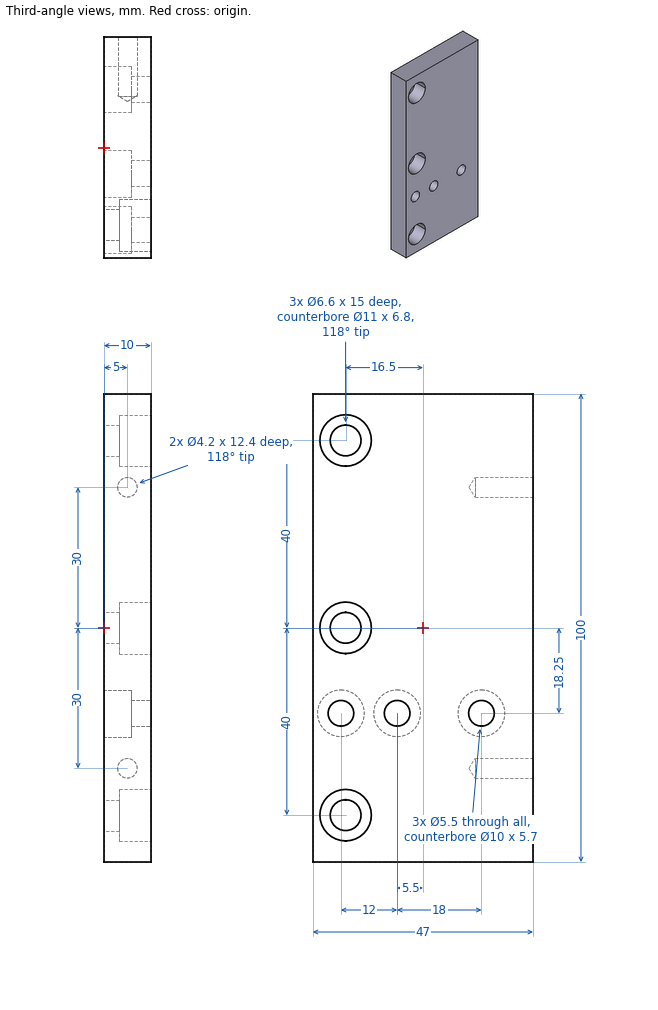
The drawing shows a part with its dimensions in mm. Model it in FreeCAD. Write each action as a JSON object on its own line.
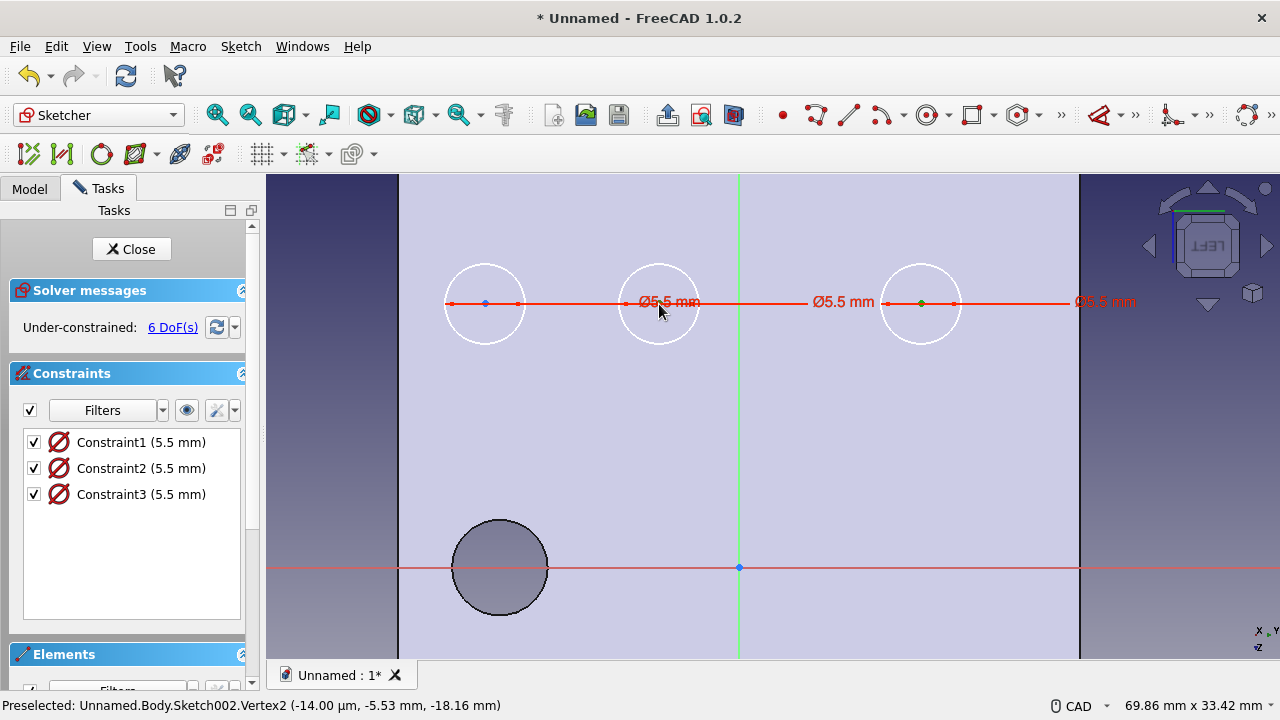
{"action": "key", "text": "h"}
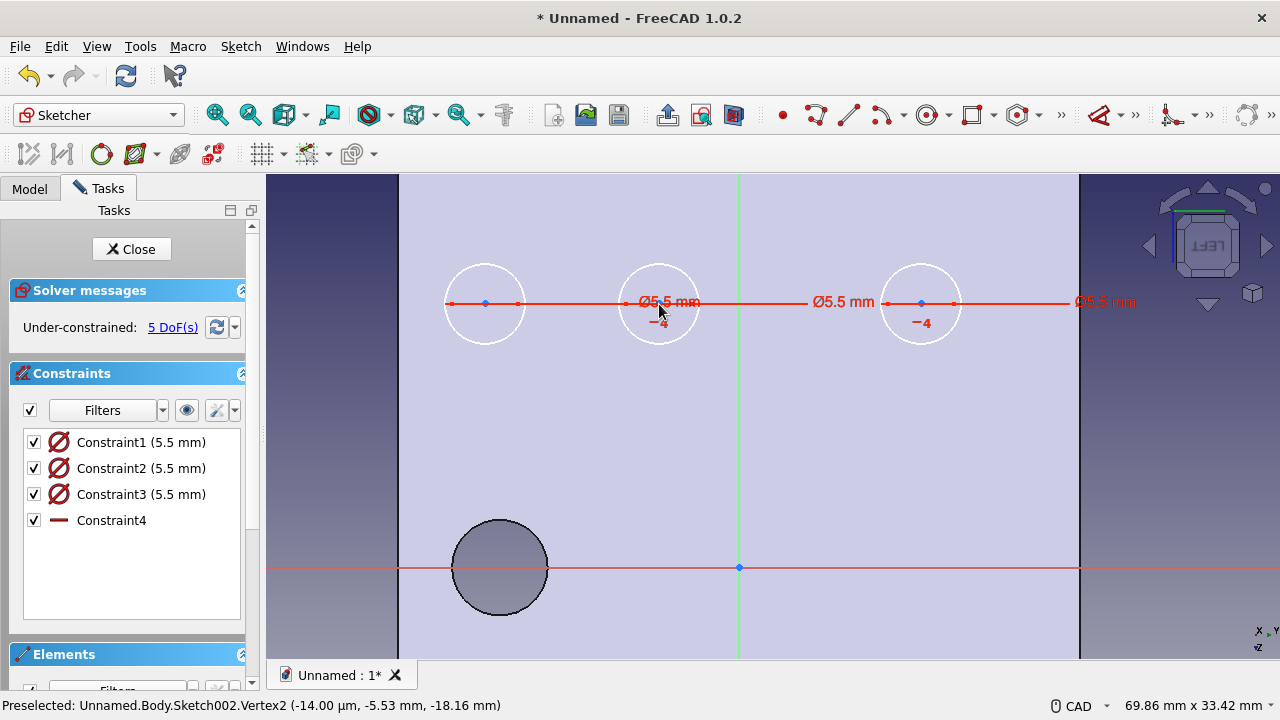
{"action": "left_click", "coordinate": [659, 304]}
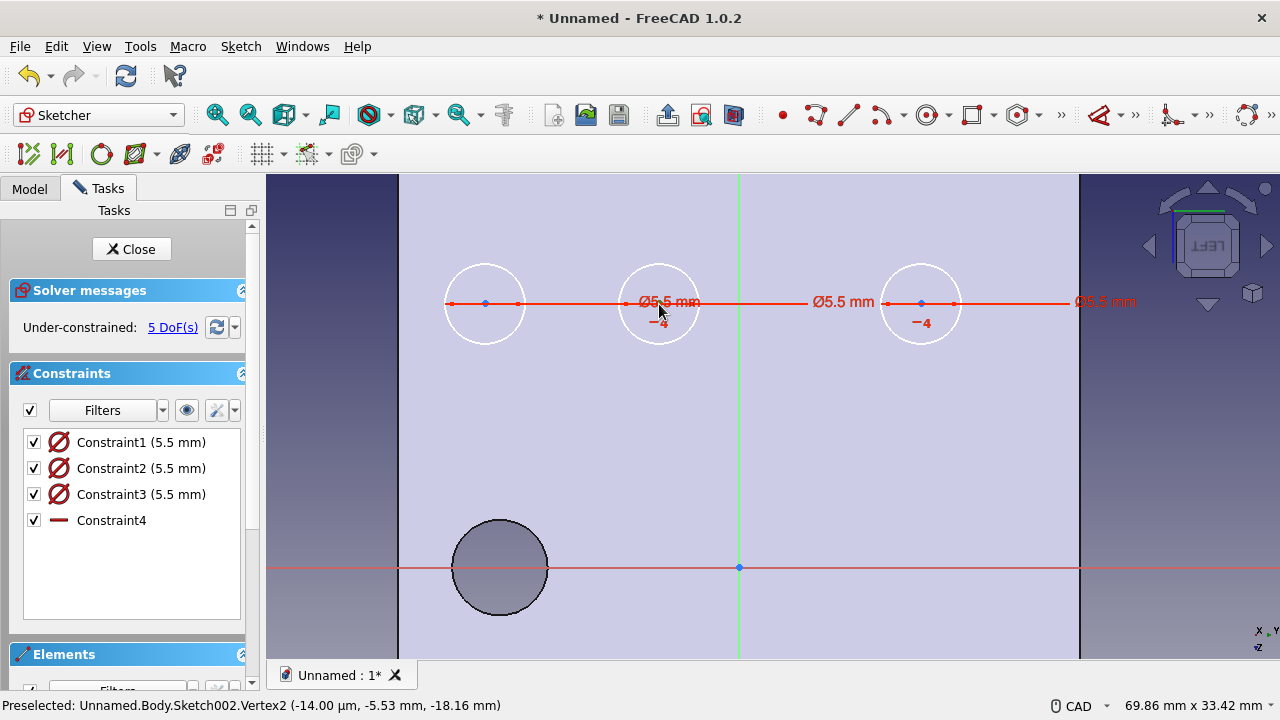
{"action": "left_click", "coordinate": [485, 304]}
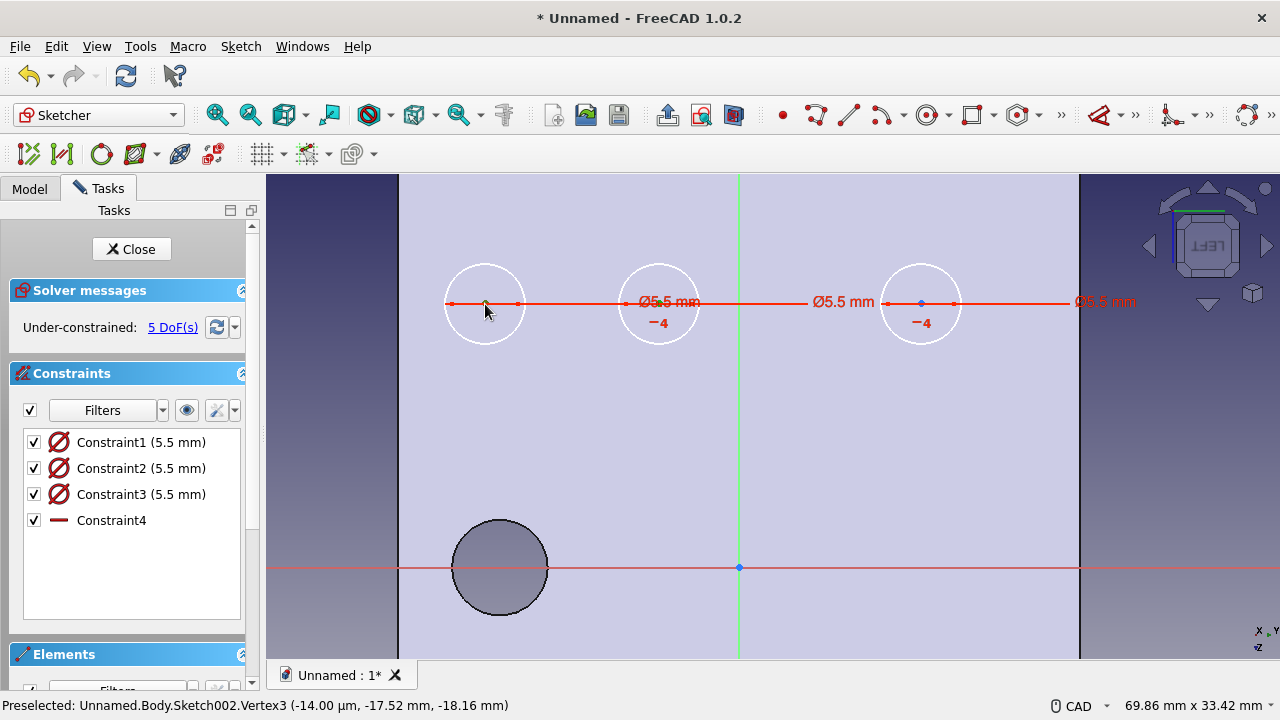
{"action": "key", "text": "h"}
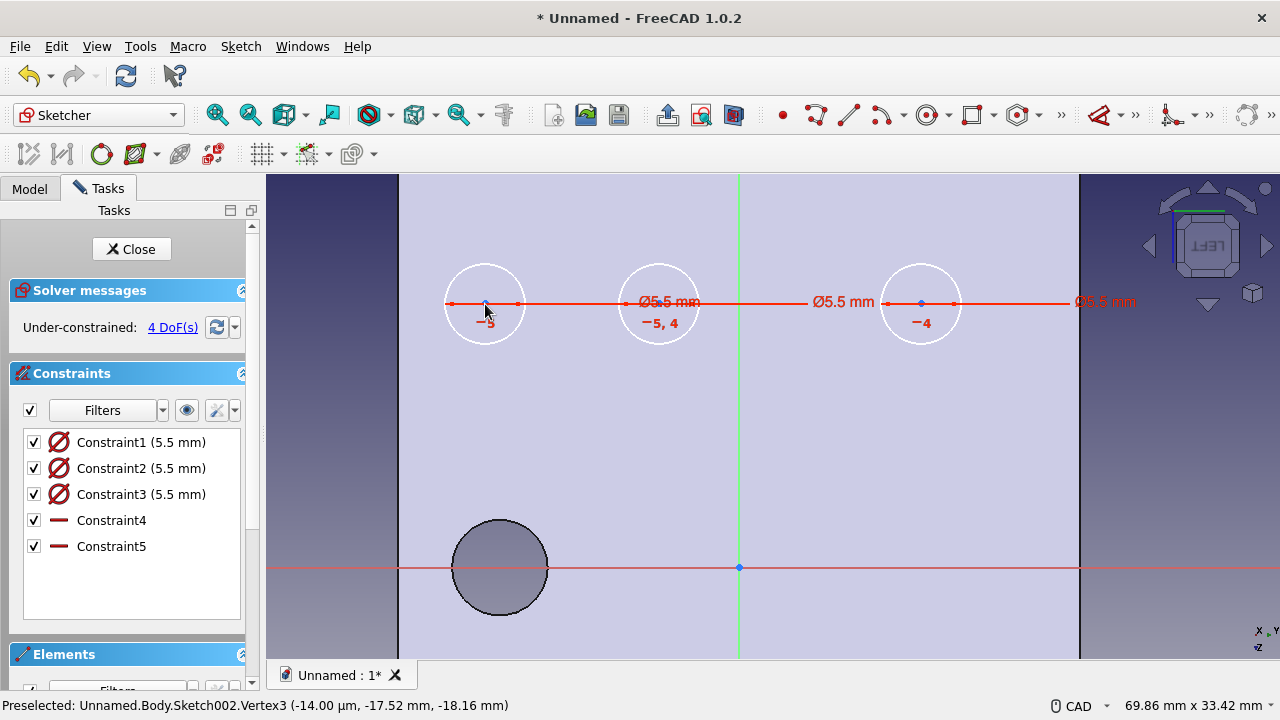
{"action": "key", "text": "d"}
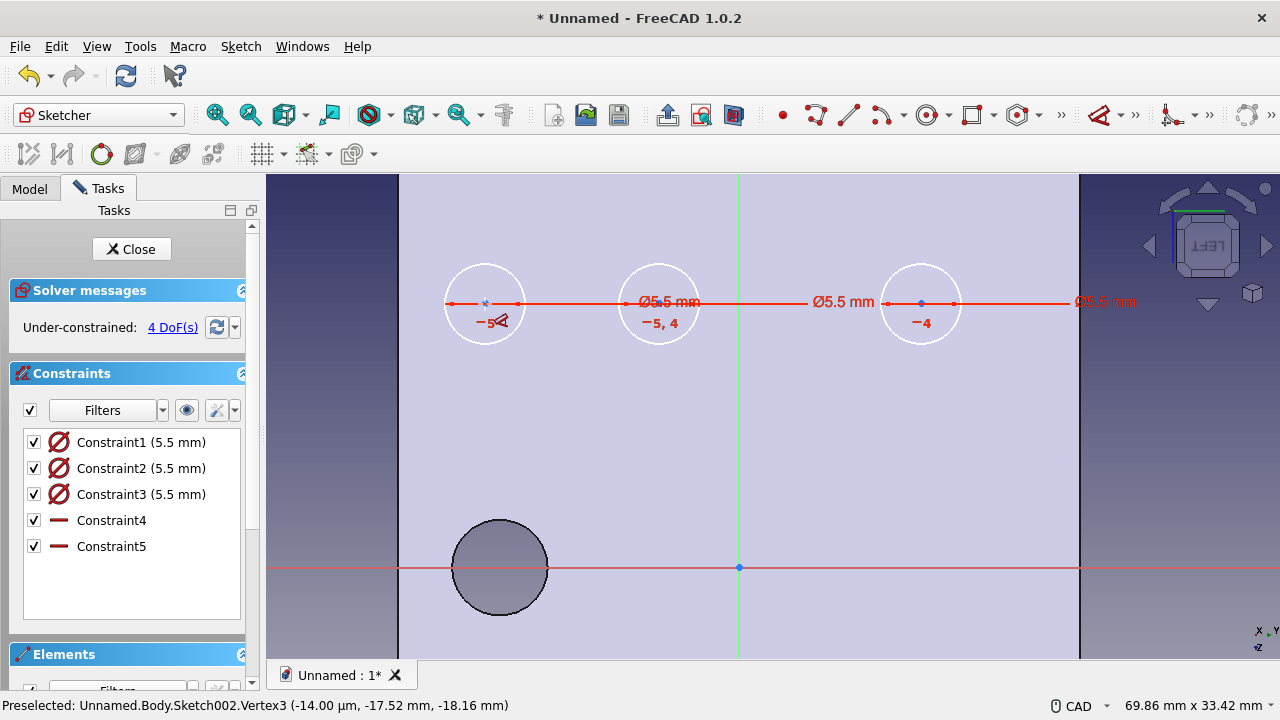
{"action": "left_click", "coordinate": [659, 304]}
{"action": "left_click", "coordinate": [699, 602]}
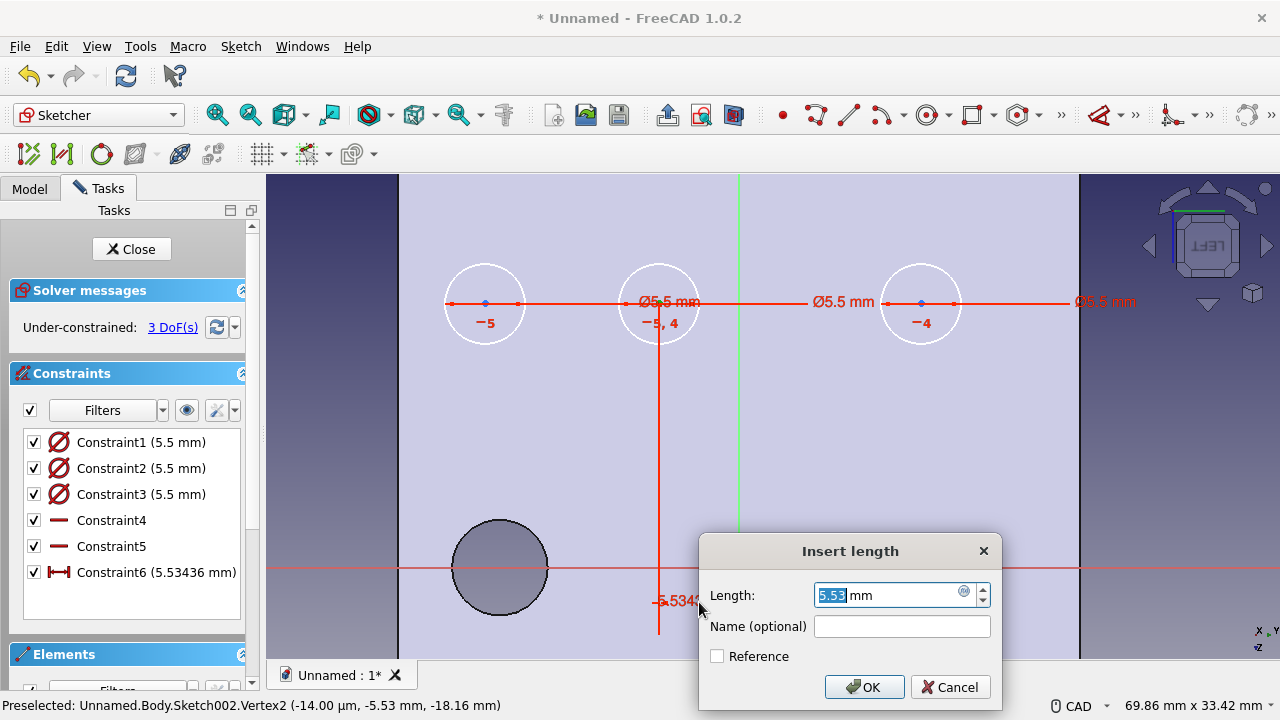
{"action": "type", "text": "5.5"}
{"action": "key", "text": "Return"}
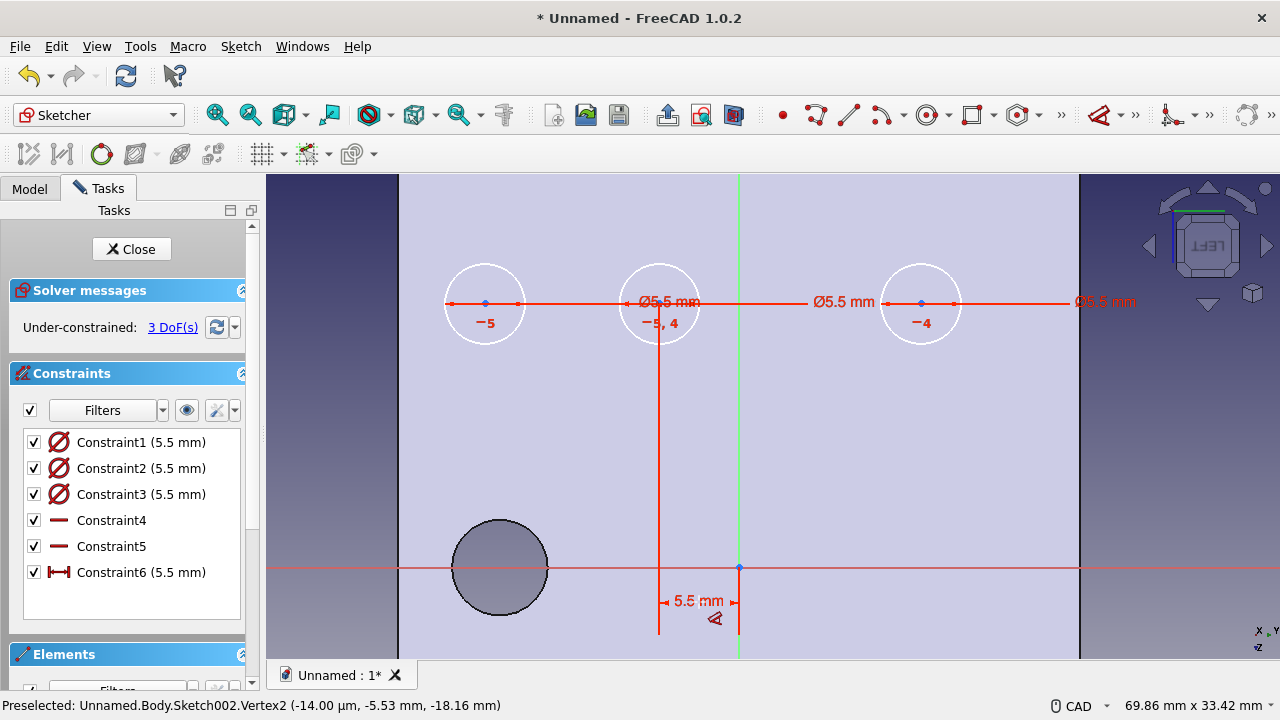
{"action": "left_click", "coordinate": [921, 304]}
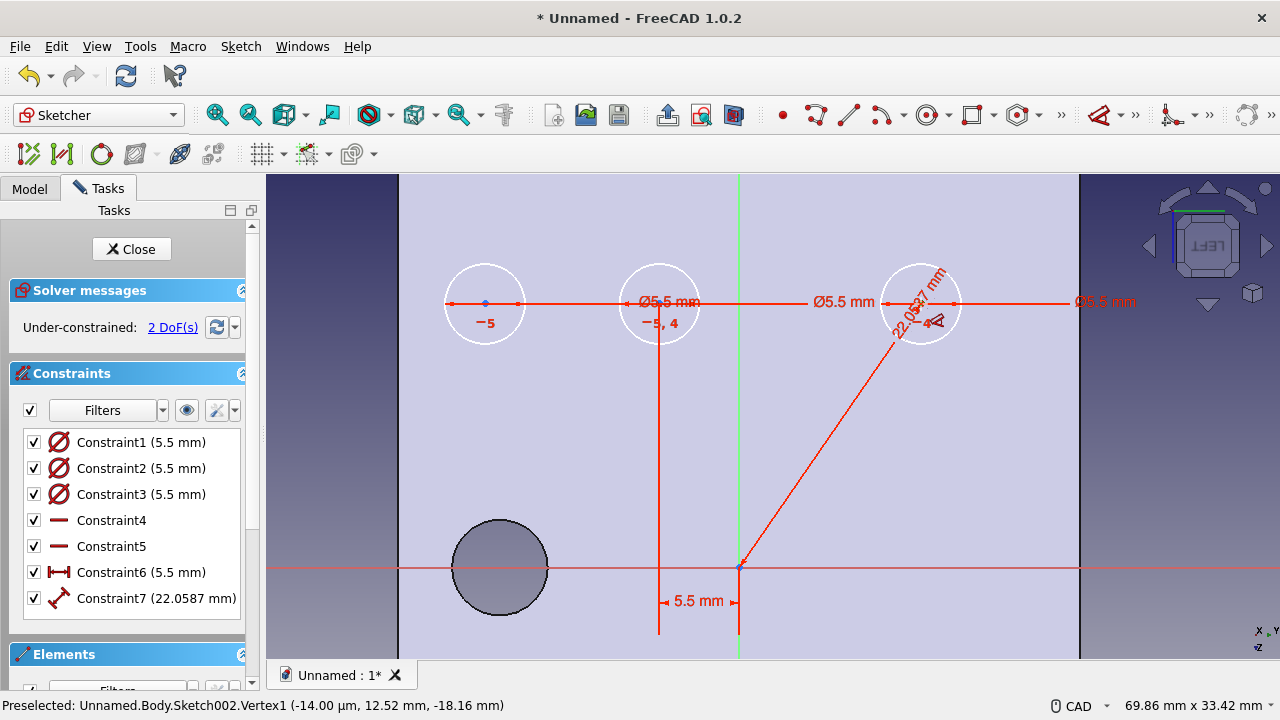
{"action": "left_click", "coordinate": [659, 304]}
{"action": "left_click", "coordinate": [790, 270]}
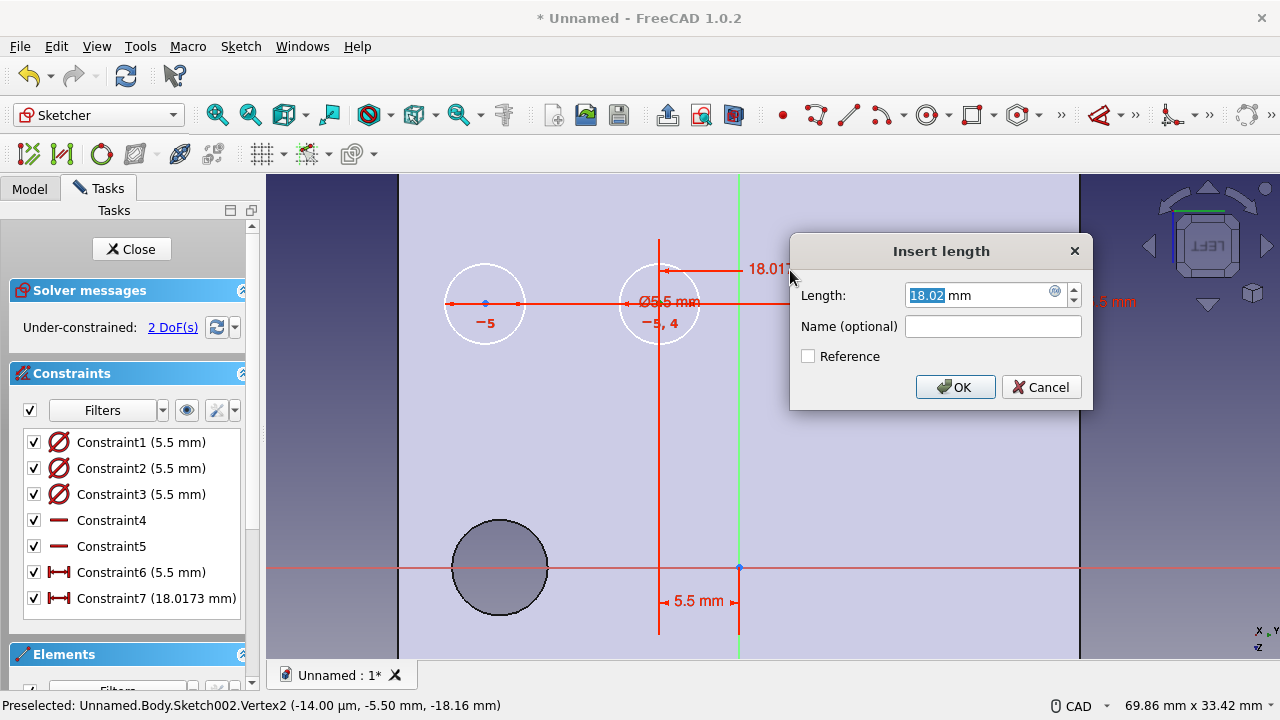
{"action": "type", "text": "18"}
{"action": "key", "text": "Return"}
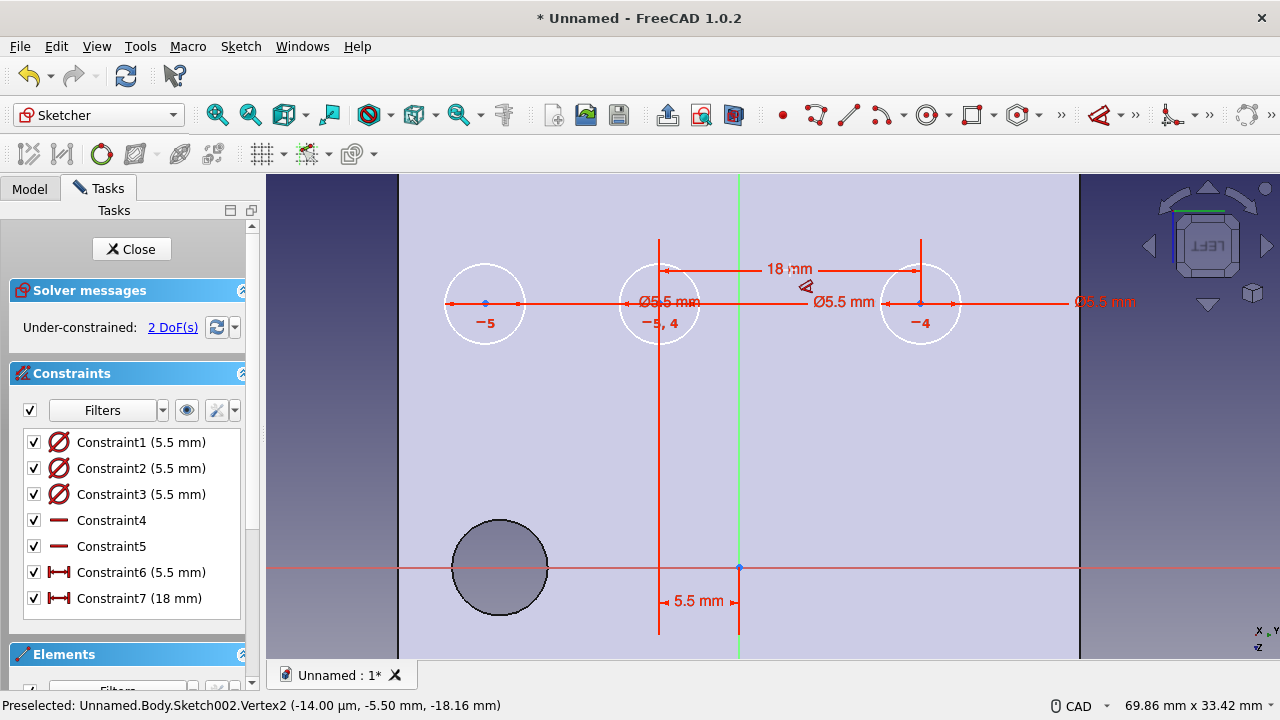
{"action": "left_click", "coordinate": [659, 304]}